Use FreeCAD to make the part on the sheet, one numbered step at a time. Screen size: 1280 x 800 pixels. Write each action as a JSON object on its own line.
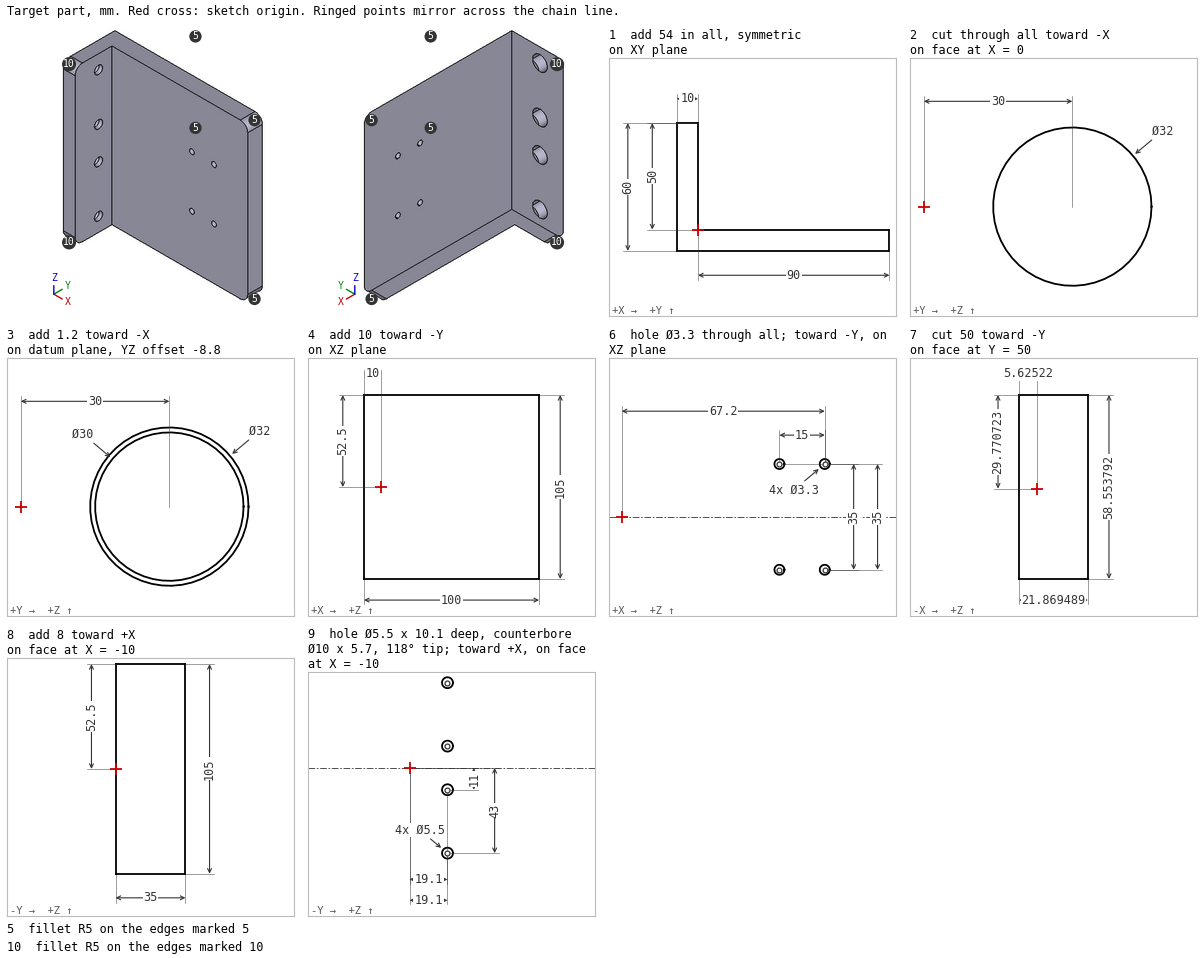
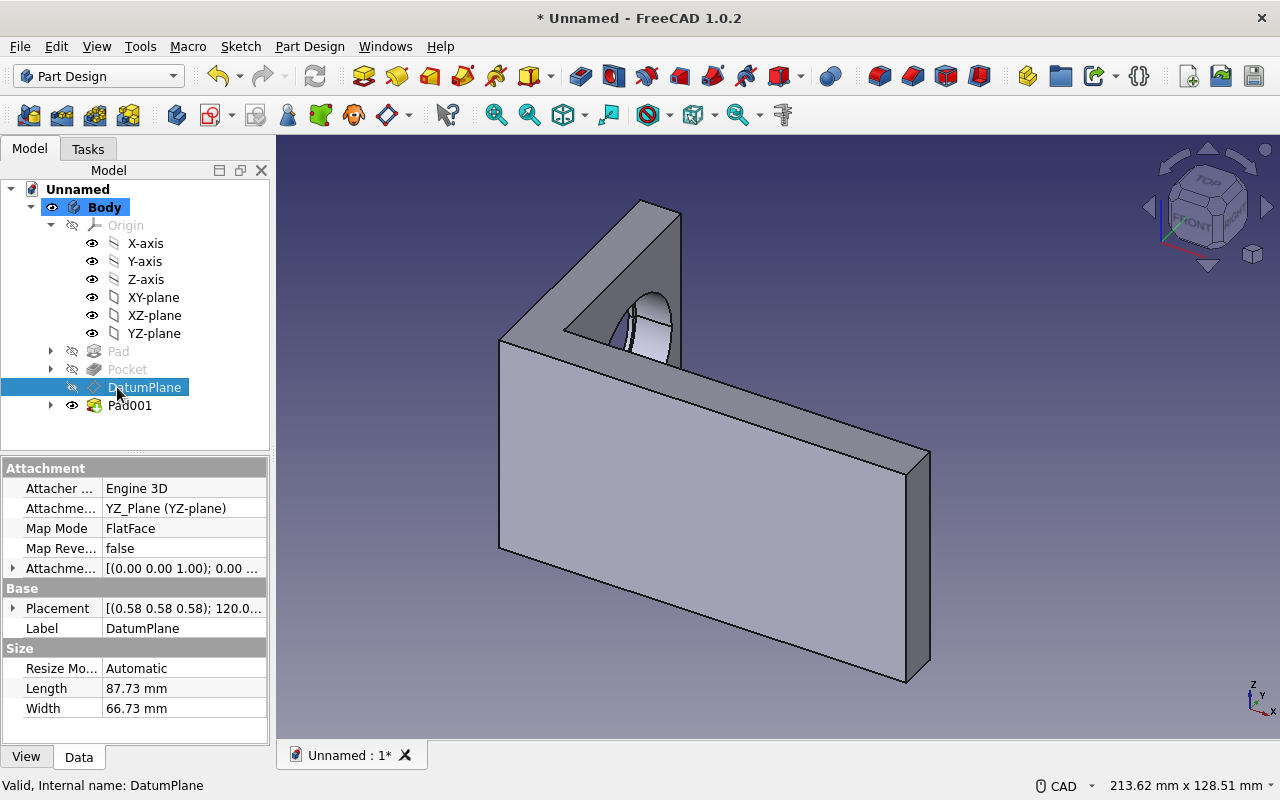
{"action": "left_click", "coordinate": [316, 699]}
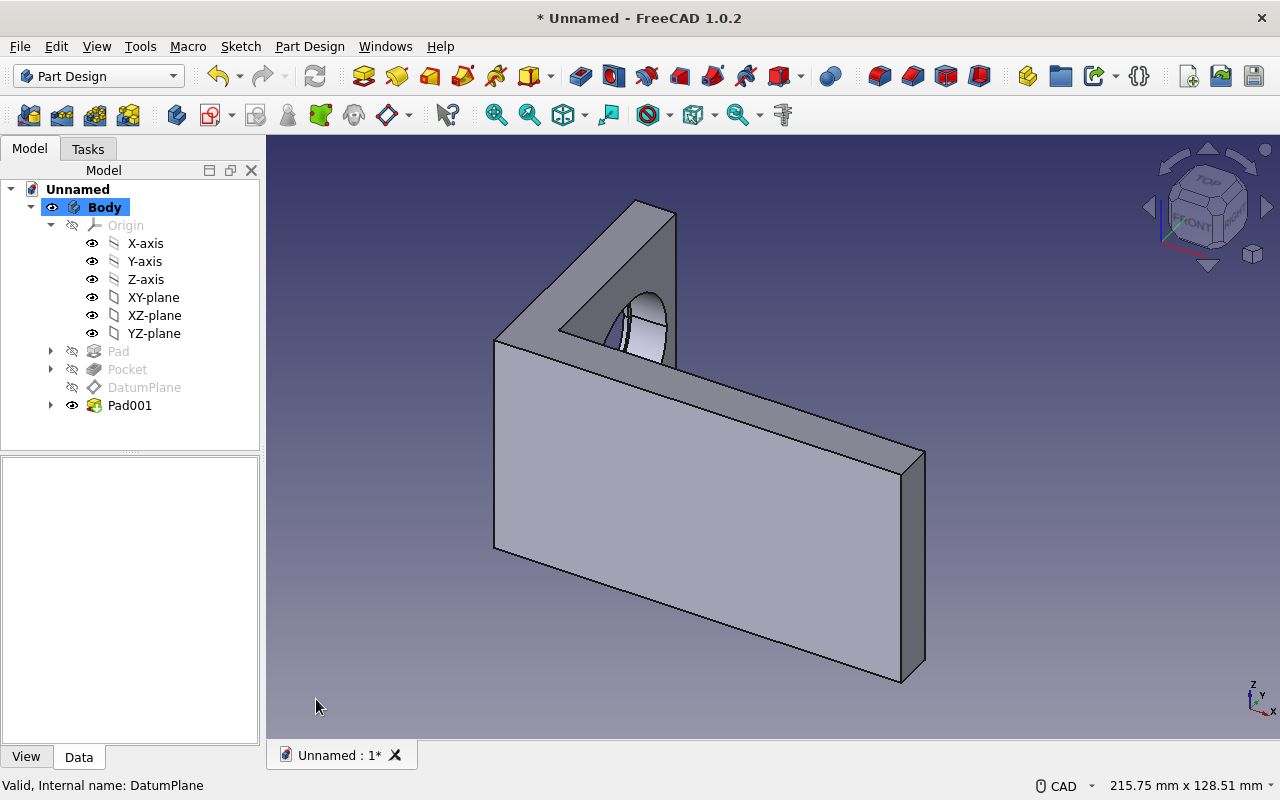
{"action": "left_click", "coordinate": [210, 116]}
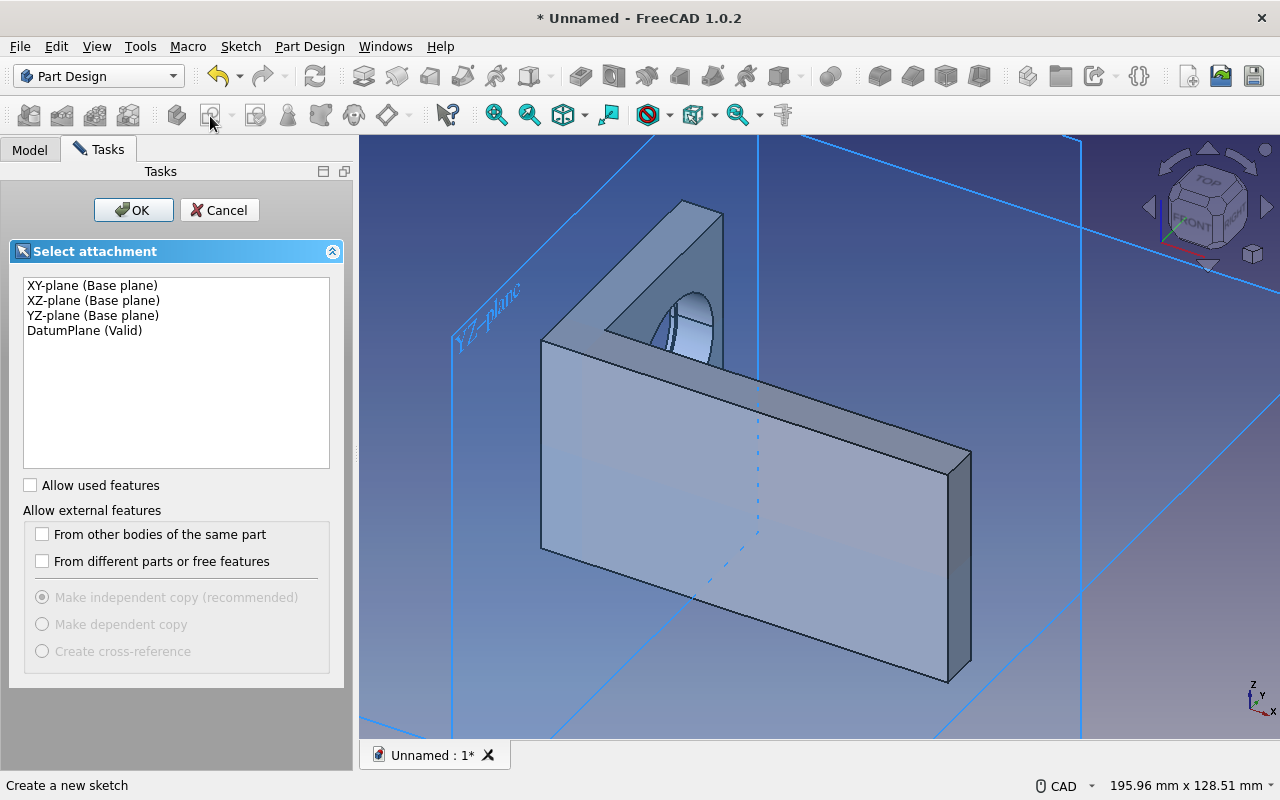
{"action": "left_click", "coordinate": [84, 300]}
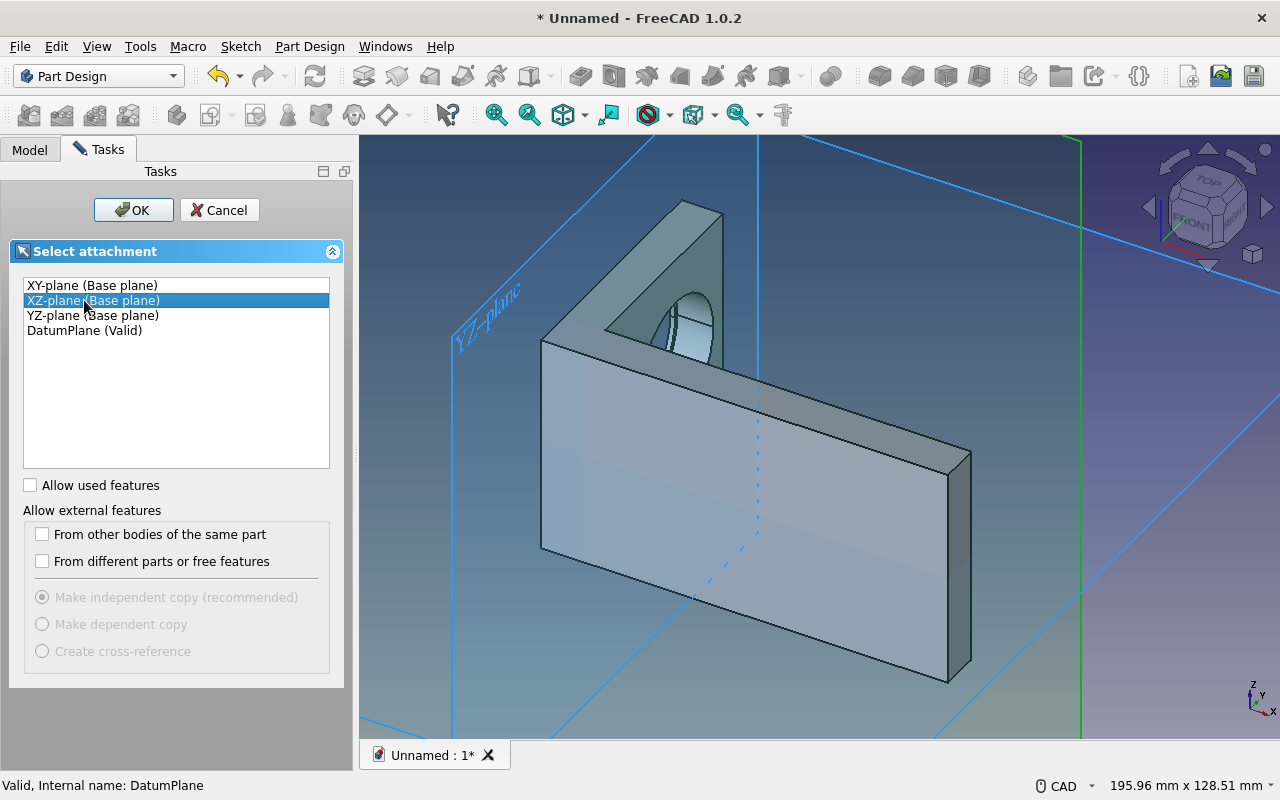
{"action": "left_click", "coordinate": [134, 210]}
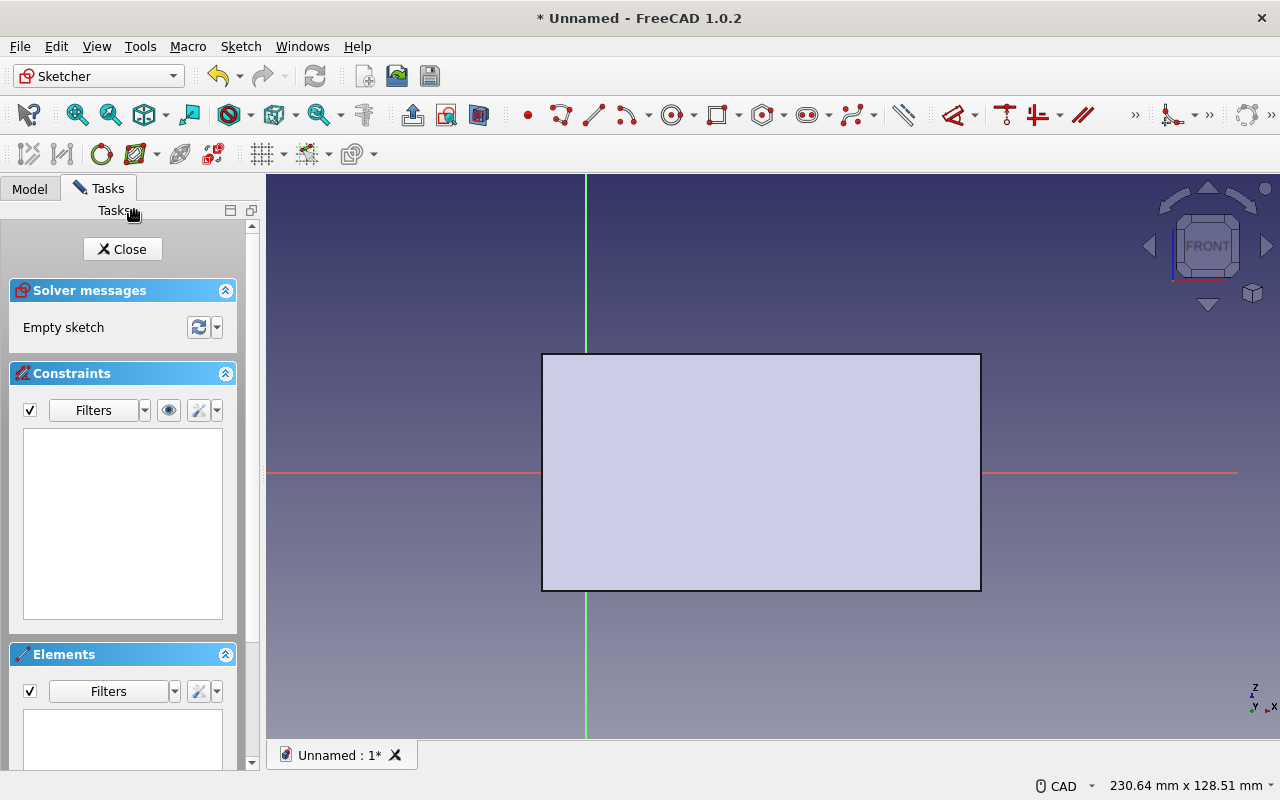
{"action": "left_click", "coordinate": [479, 116]}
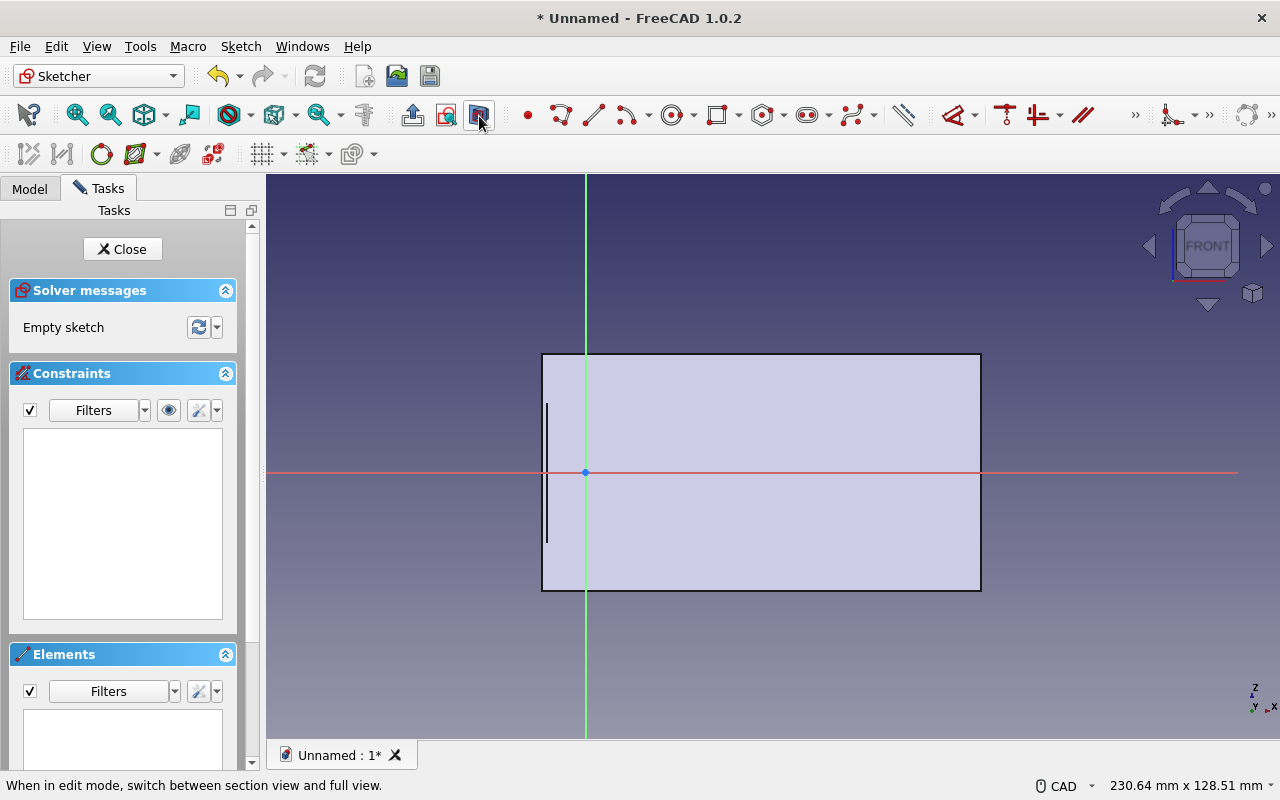
{"action": "scroll", "coordinate": [447, 384], "scroll_direction": "down", "scroll_amount": 1}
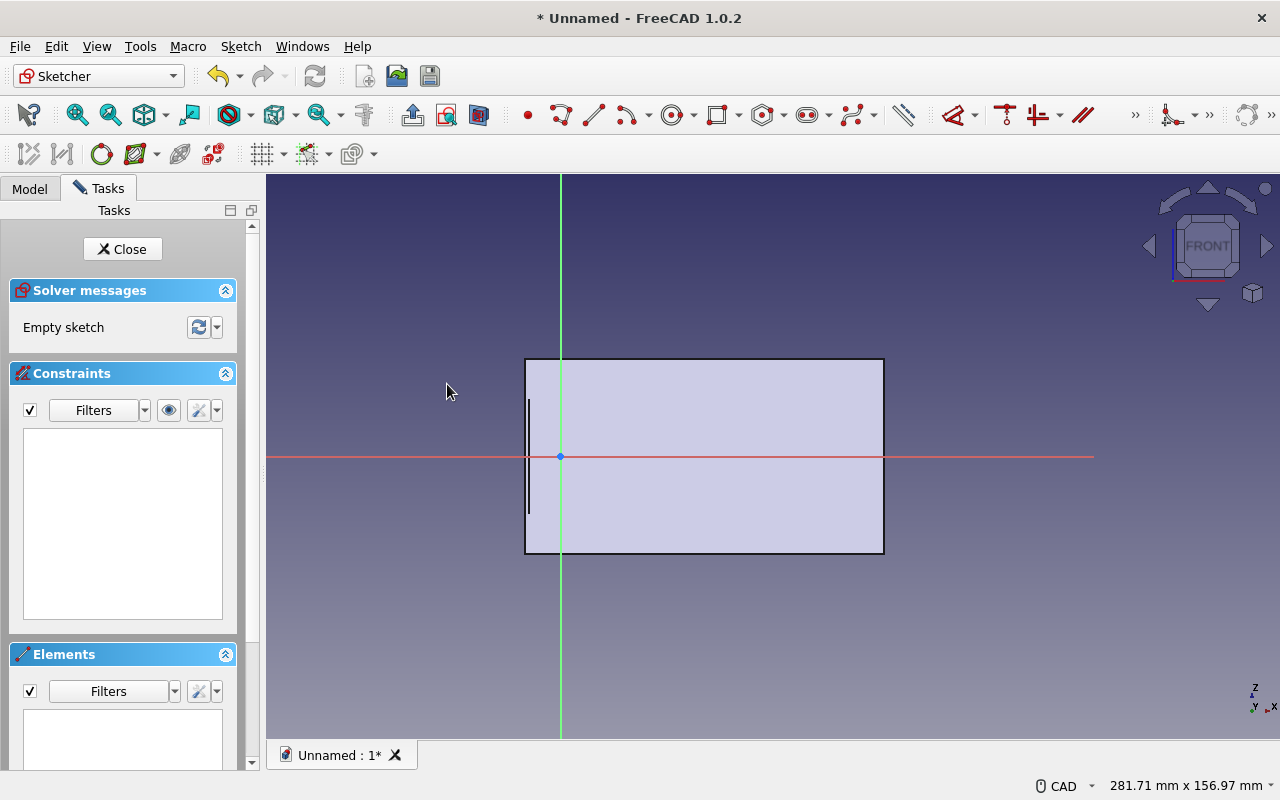
{"action": "left_click", "coordinate": [716, 116]}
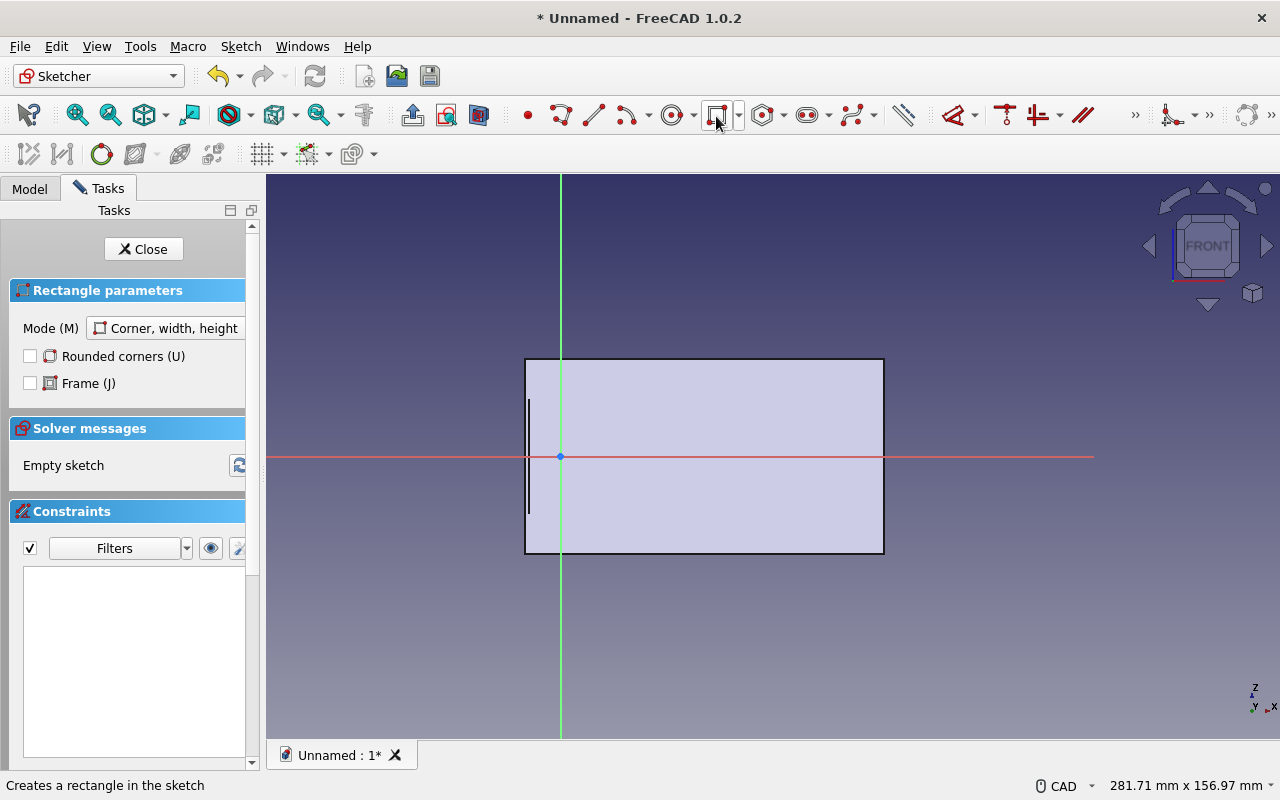
{"action": "left_click", "coordinate": [525, 268]}
{"action": "mouse_move", "coordinate": [884, 646]}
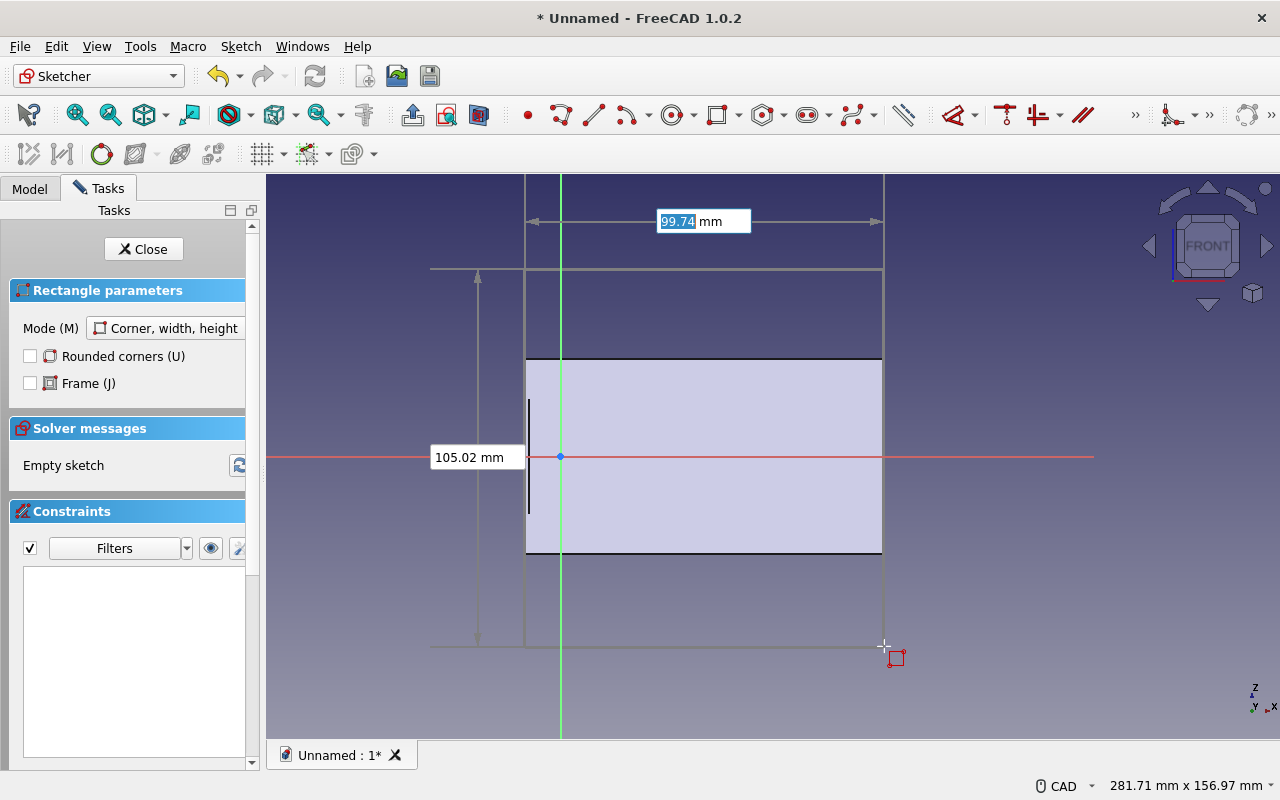
{"action": "type", "text": "100"}
{"action": "key", "text": "Tab"}
{"action": "type", "text": "105"}
{"action": "key", "text": "Return"}
{"action": "key", "text": "Escape"}